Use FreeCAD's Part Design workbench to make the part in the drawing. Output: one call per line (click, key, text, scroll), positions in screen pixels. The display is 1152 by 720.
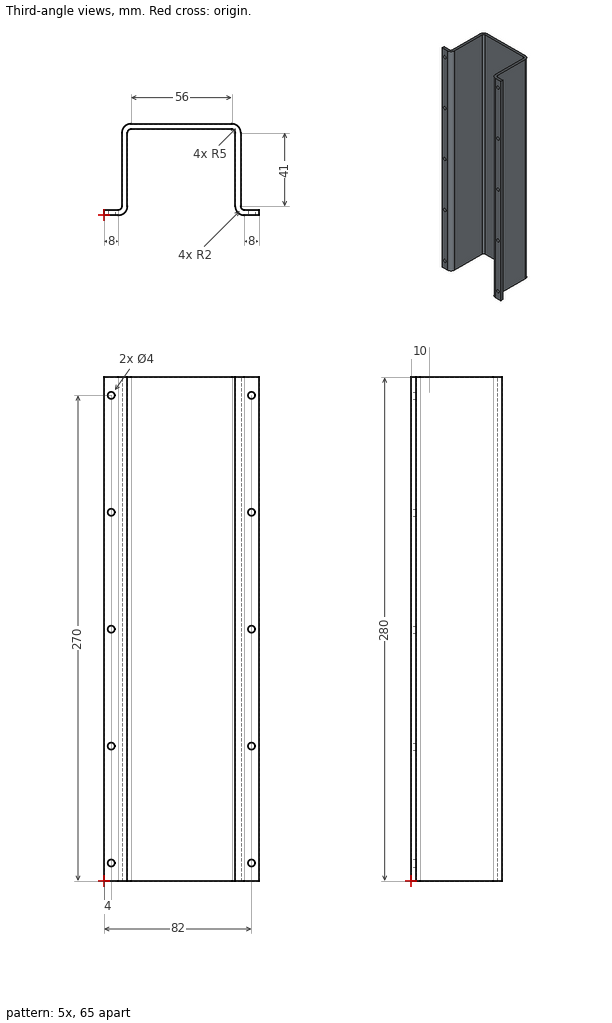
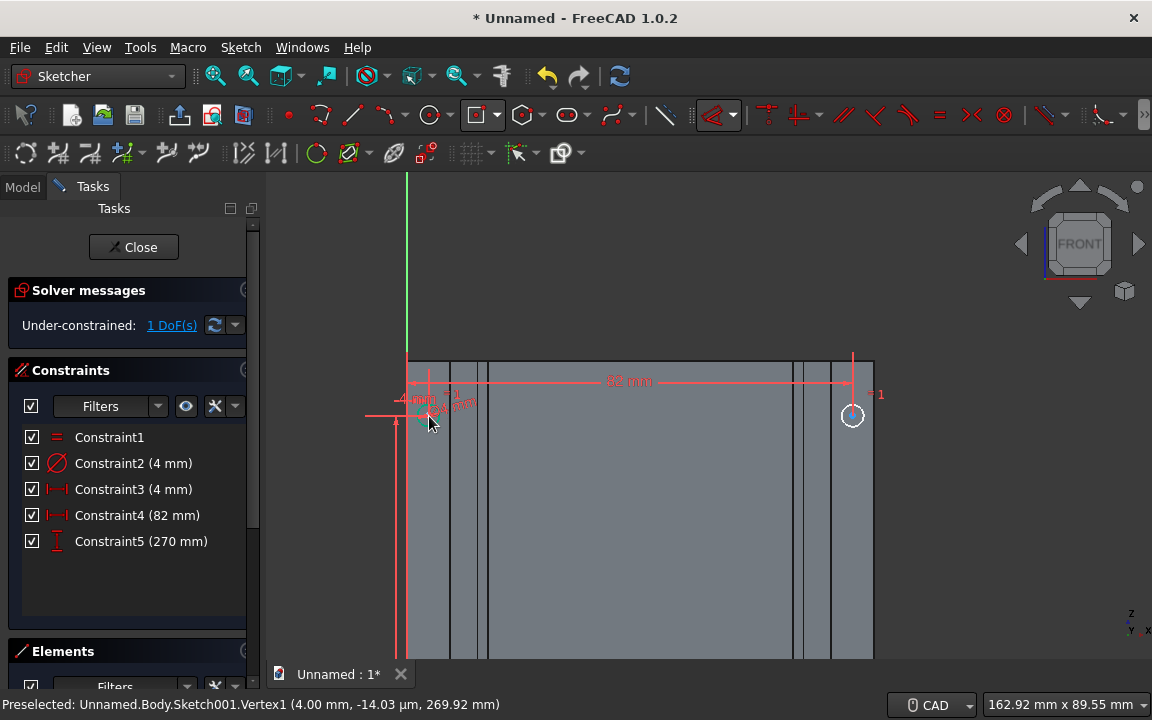
click(853, 416)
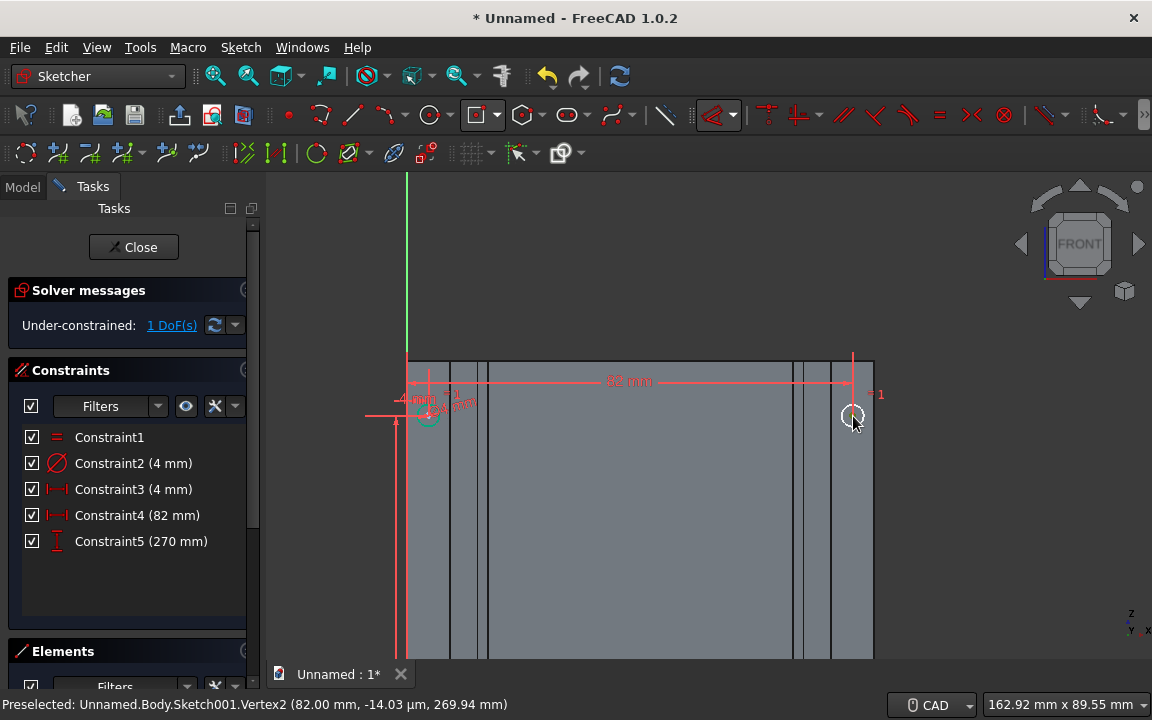
key(i)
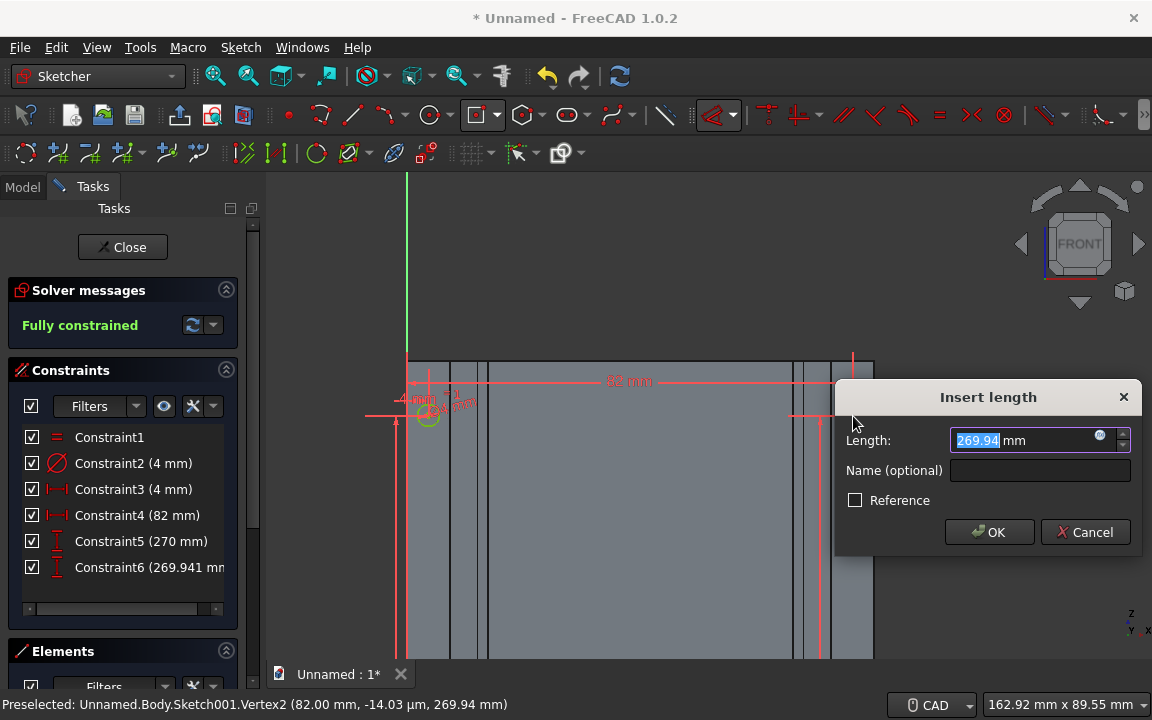
text(270)
key(Return)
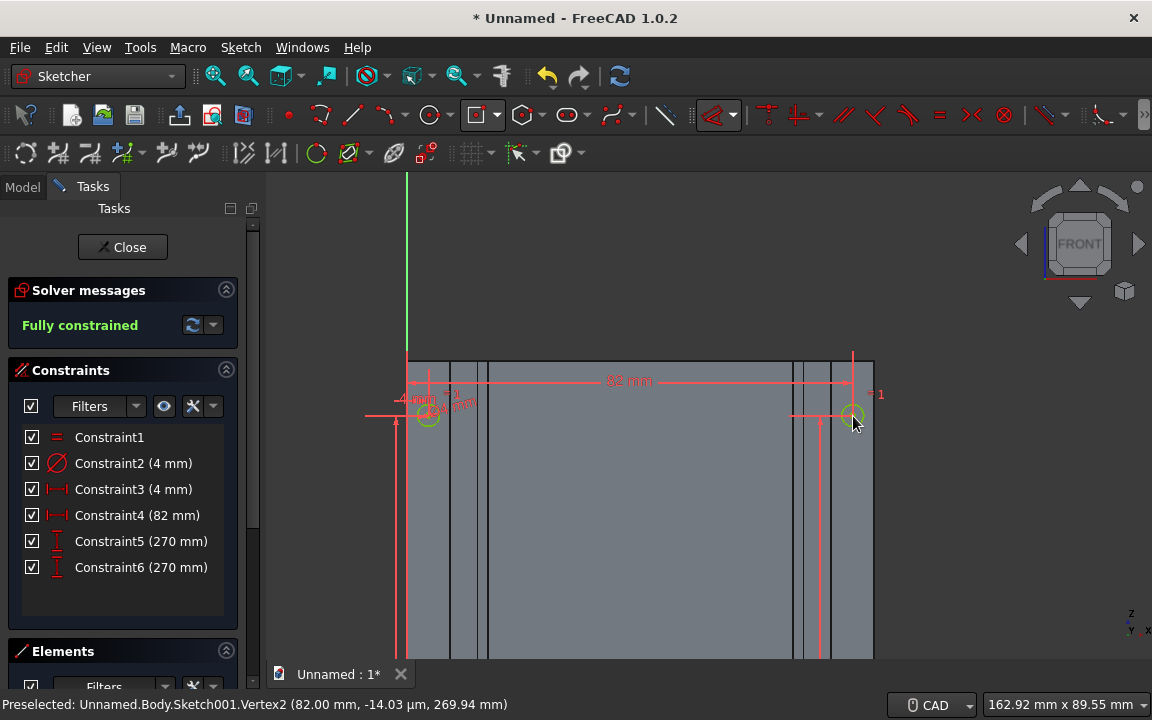
click(123, 247)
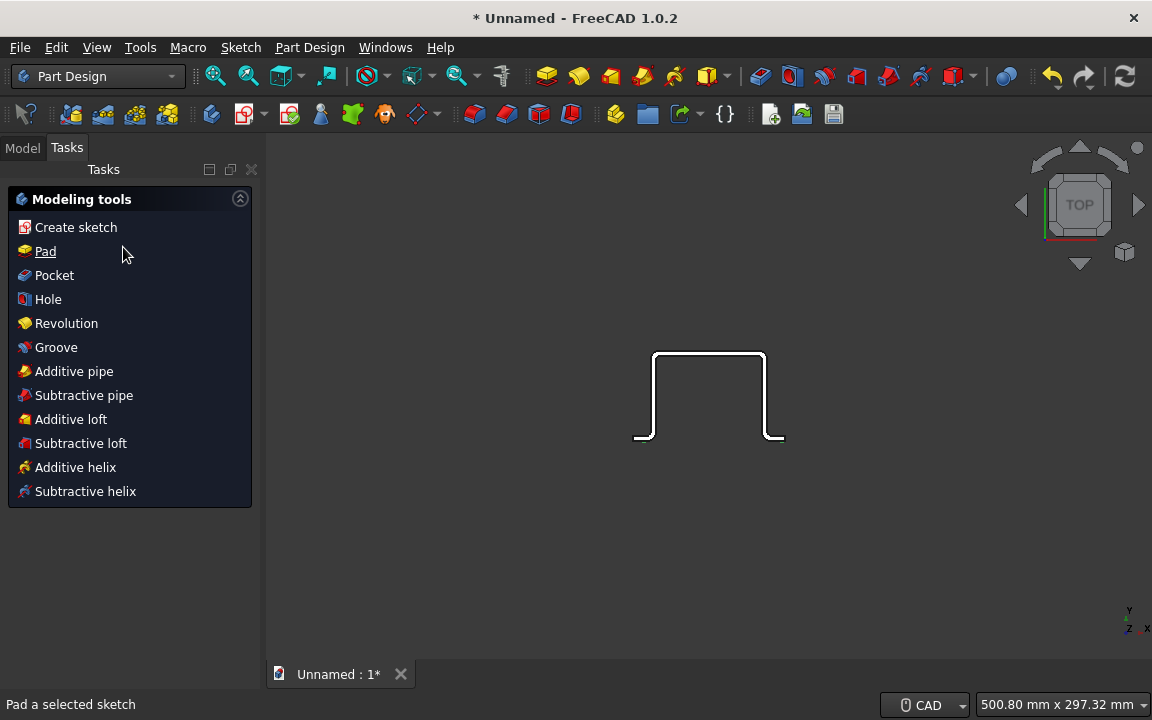
click(762, 76)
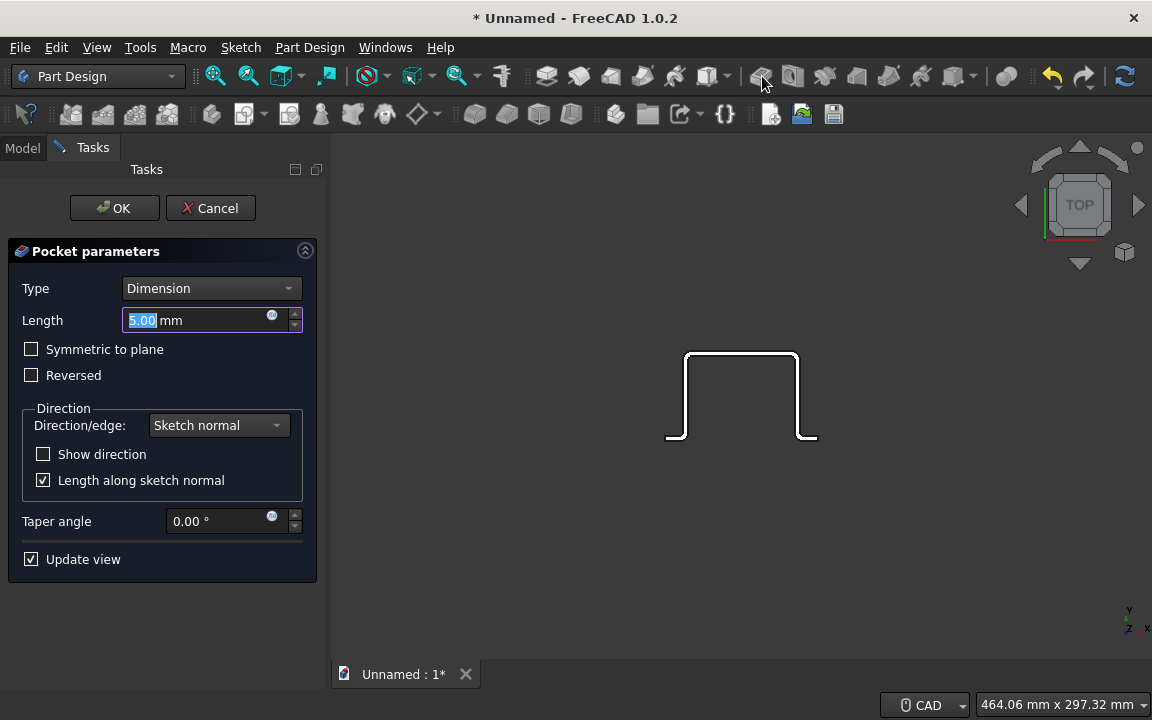
text(10)
key(Tab)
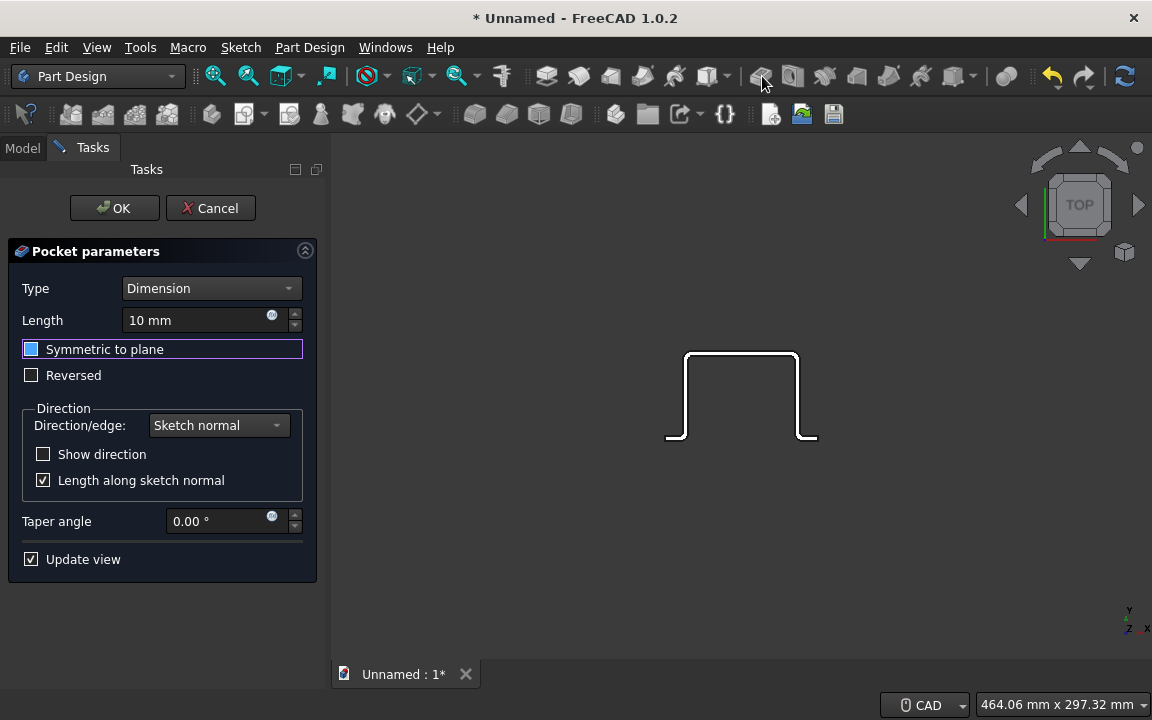
click(115, 208)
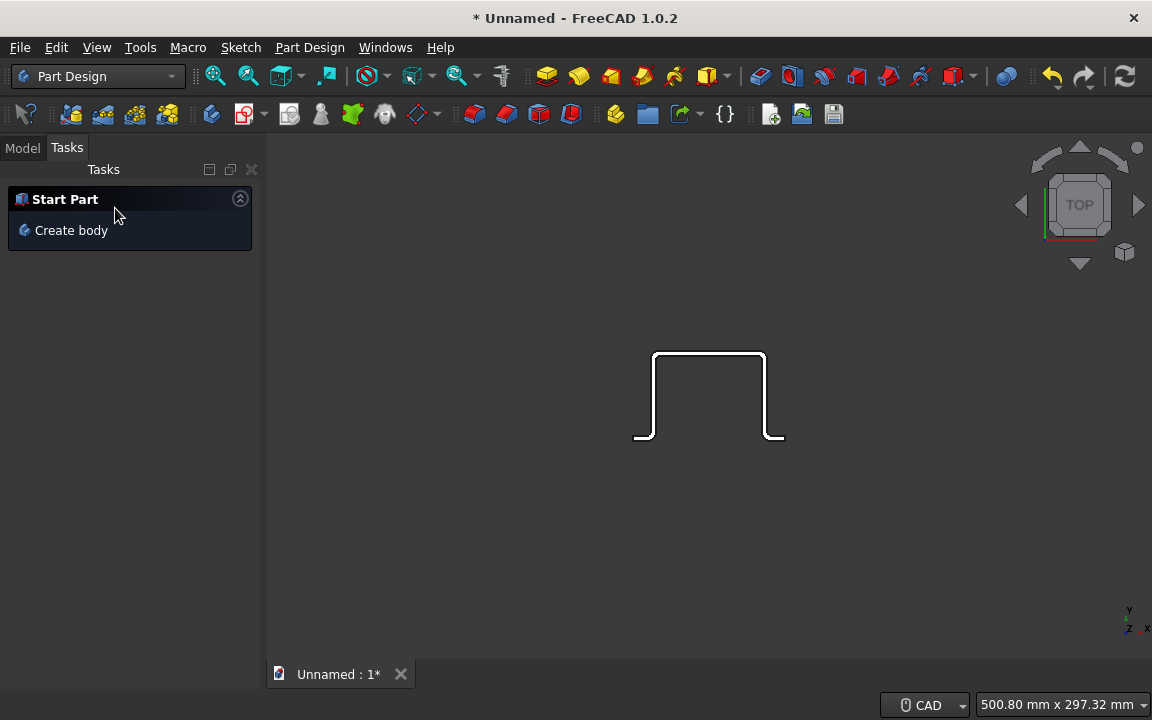
key(v)
key(f)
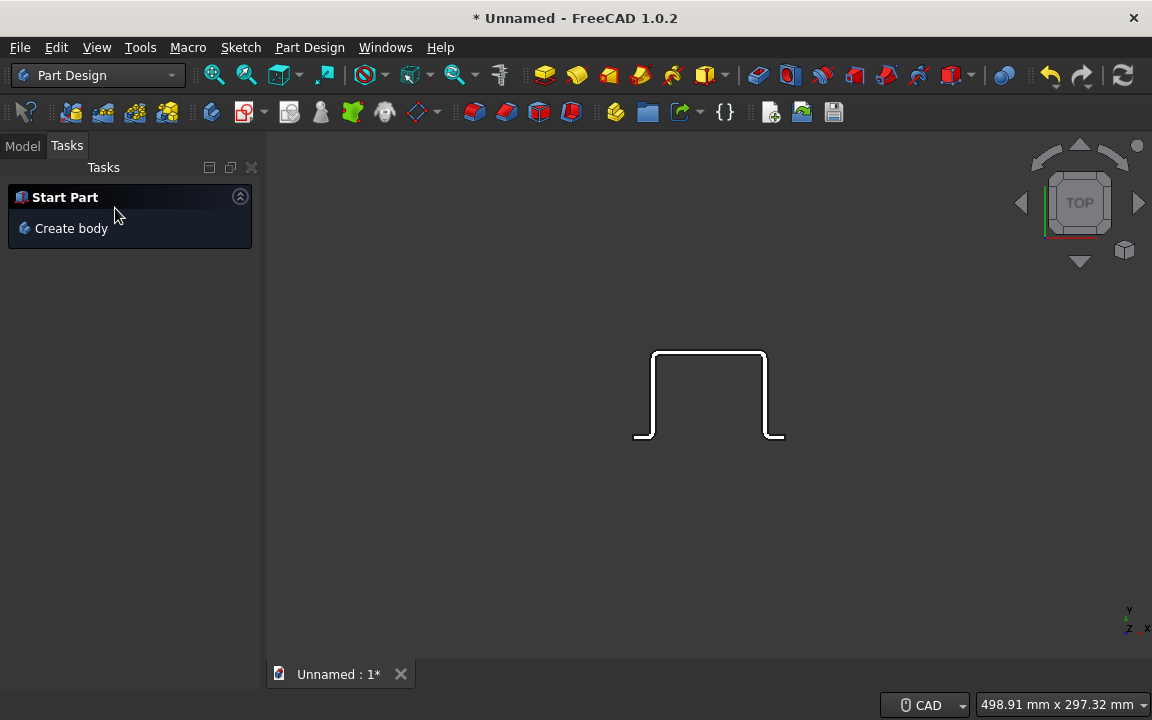
click(23, 145)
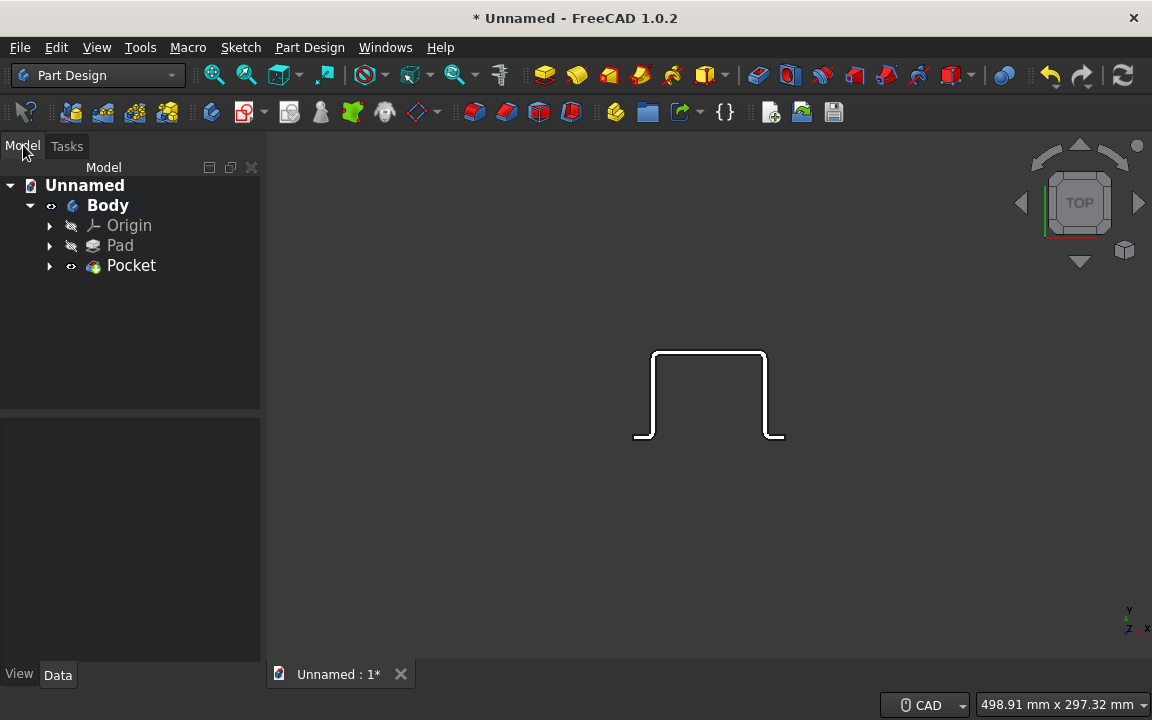
click(116, 266)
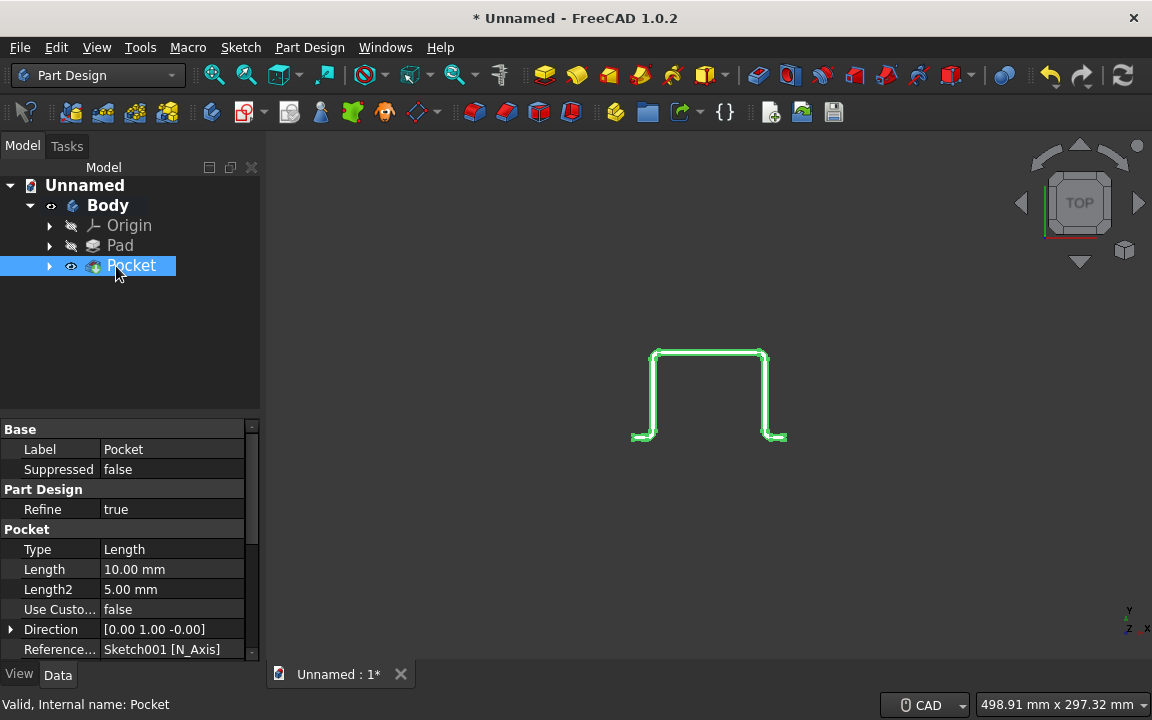
click(104, 112)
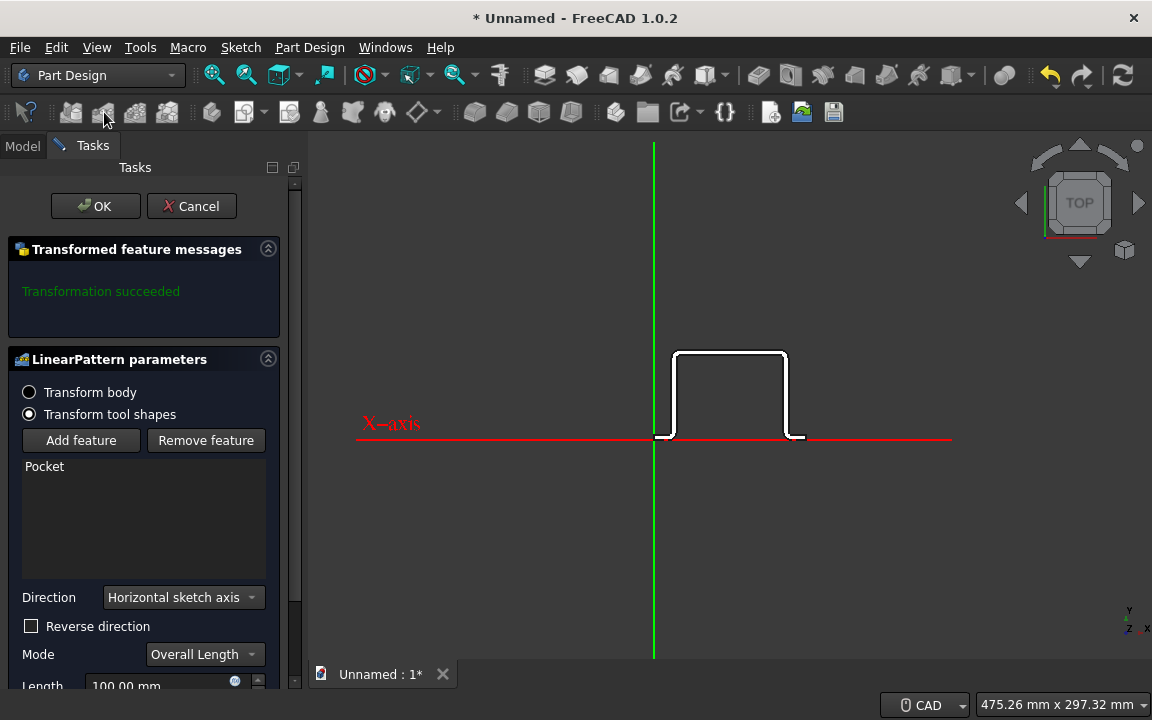
click(184, 598)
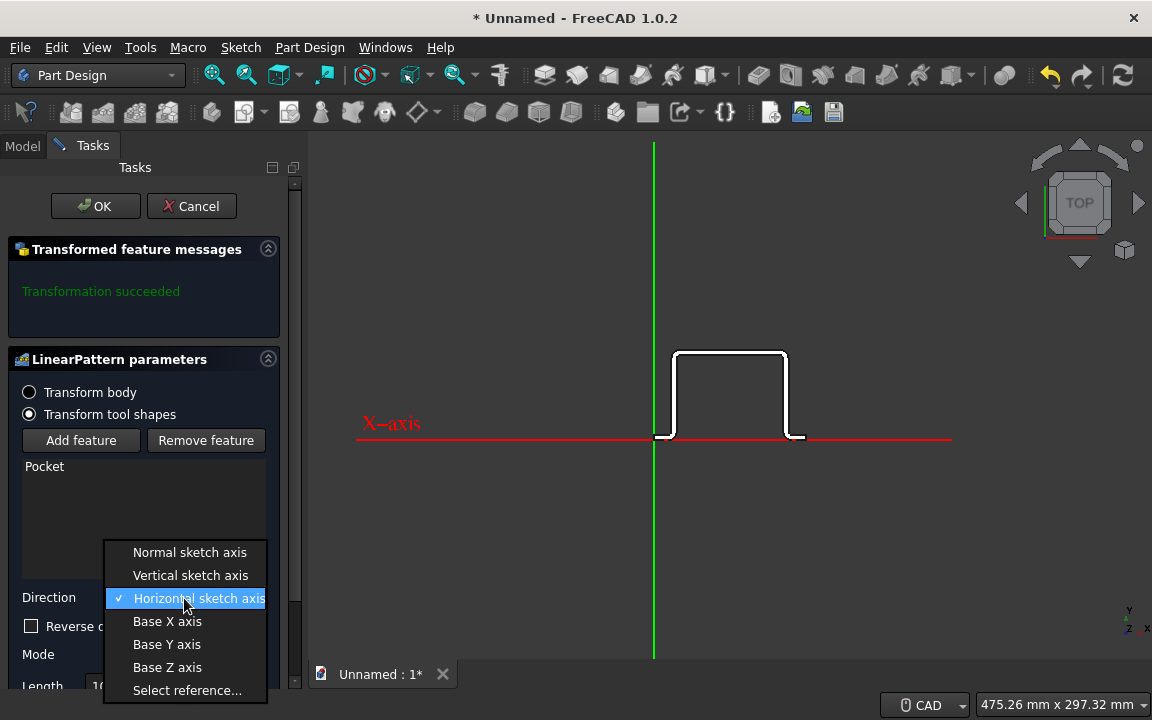
click(184, 668)